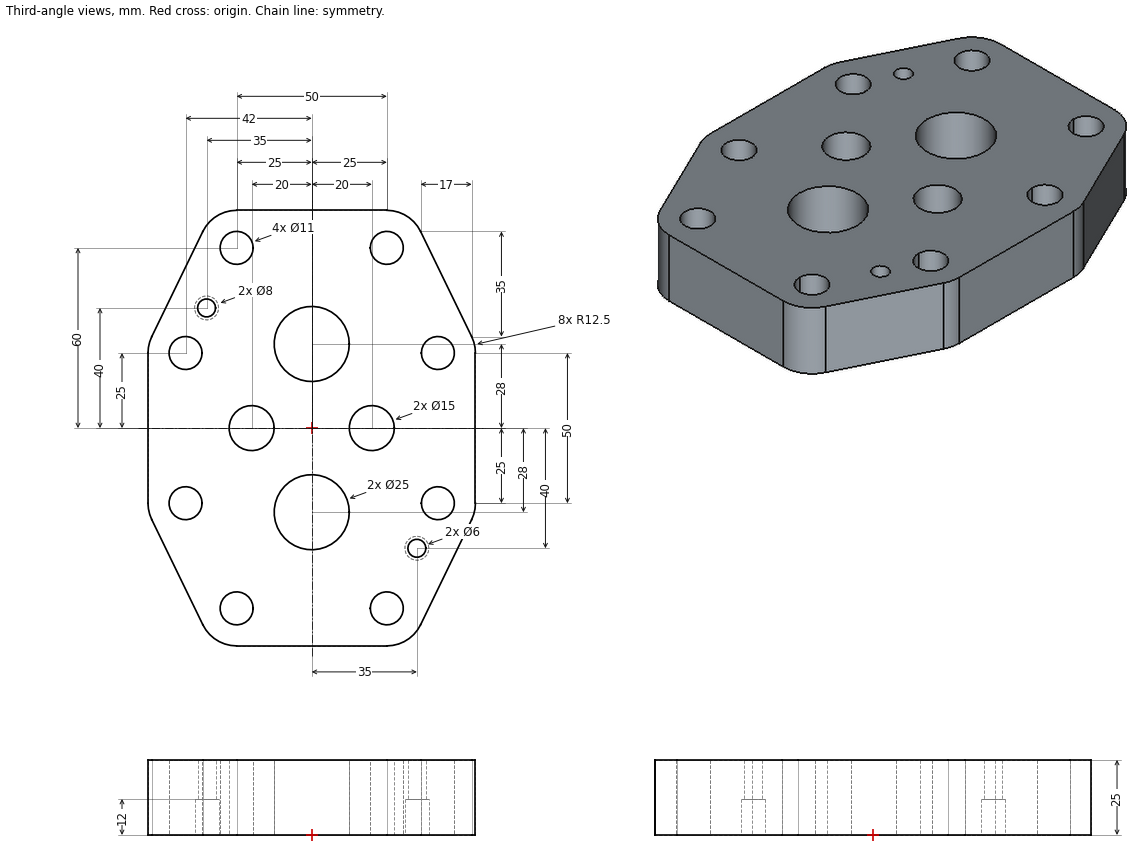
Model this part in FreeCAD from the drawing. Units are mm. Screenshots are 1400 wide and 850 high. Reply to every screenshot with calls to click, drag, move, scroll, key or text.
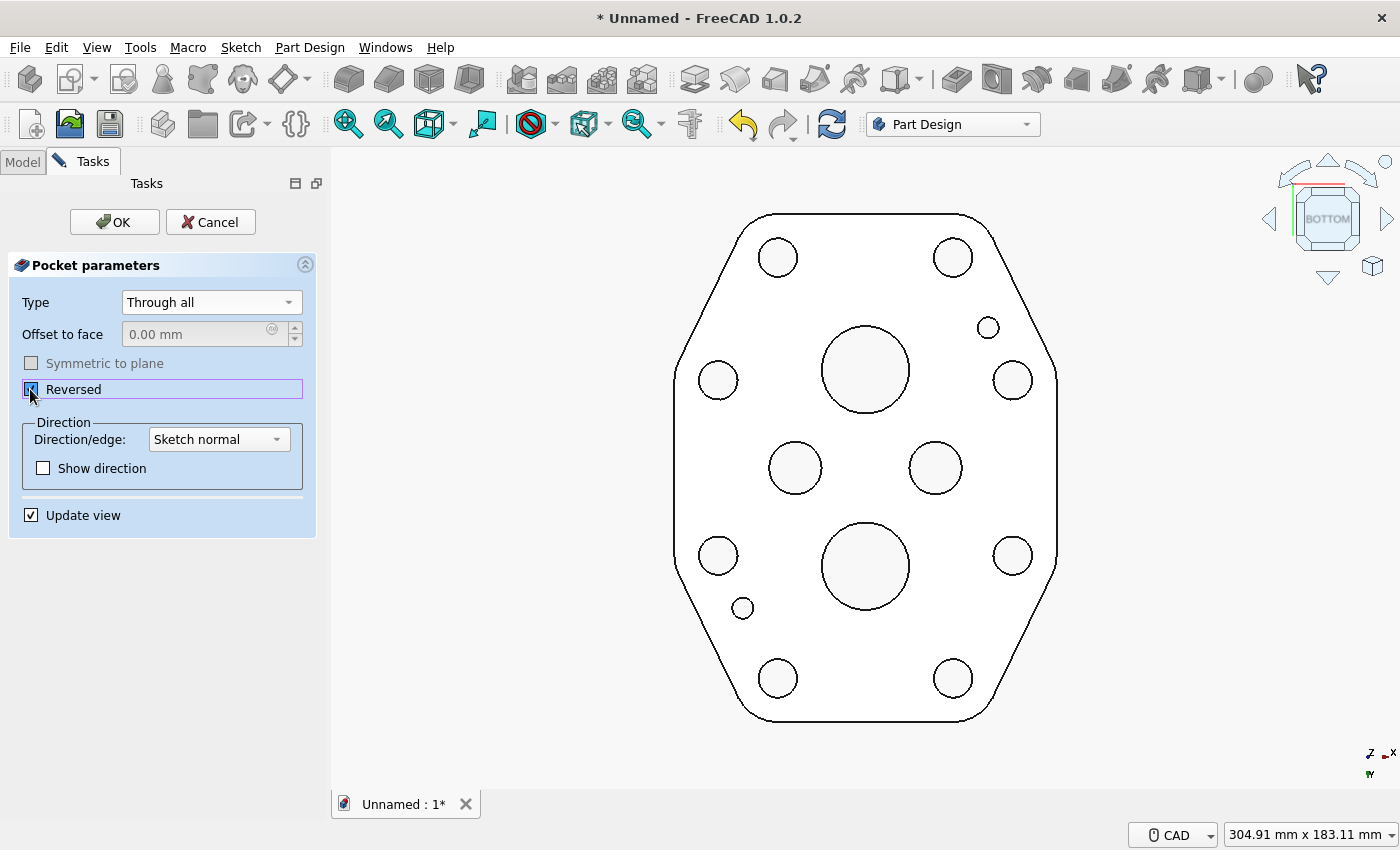
click(115, 222)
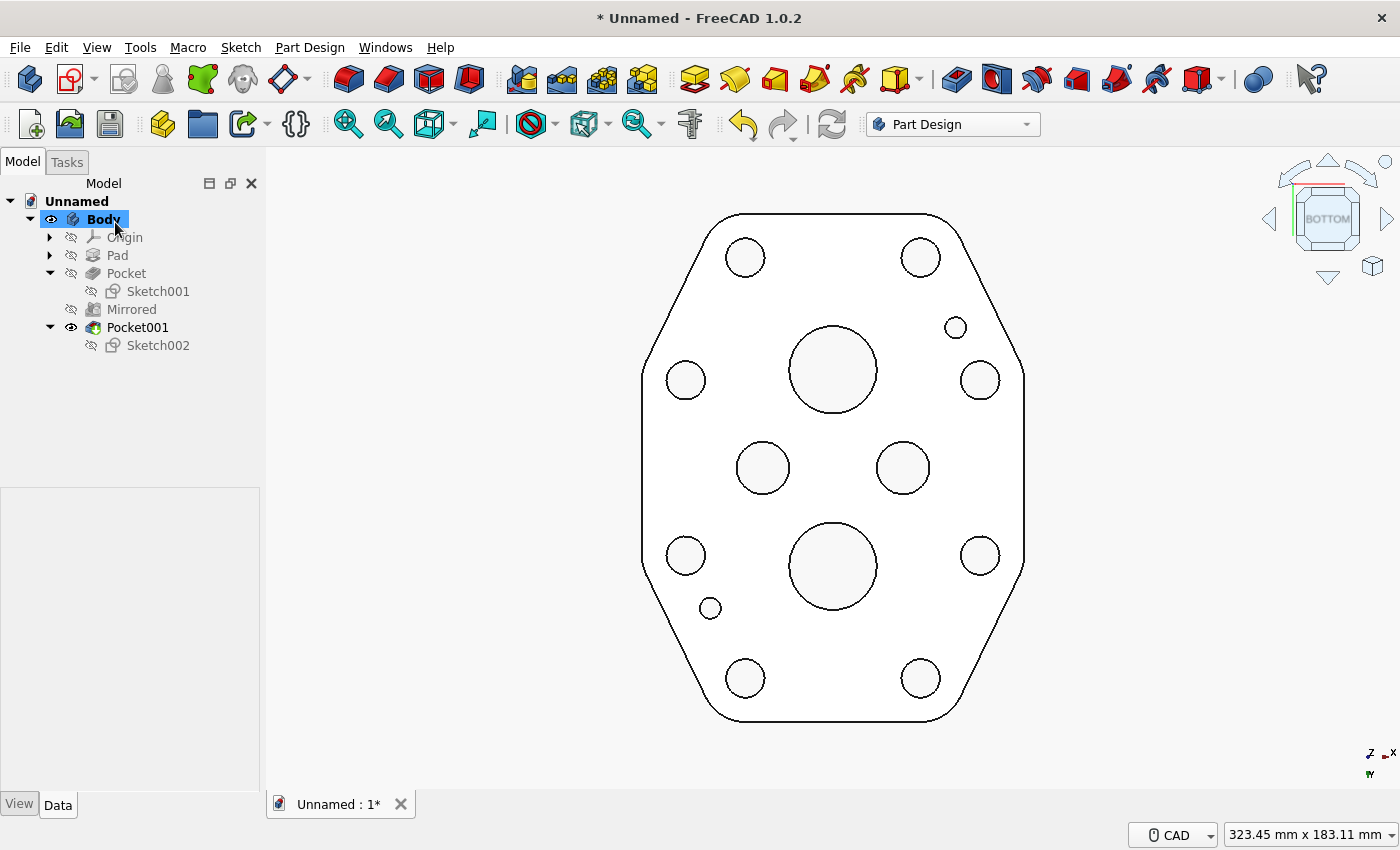
click(724, 322)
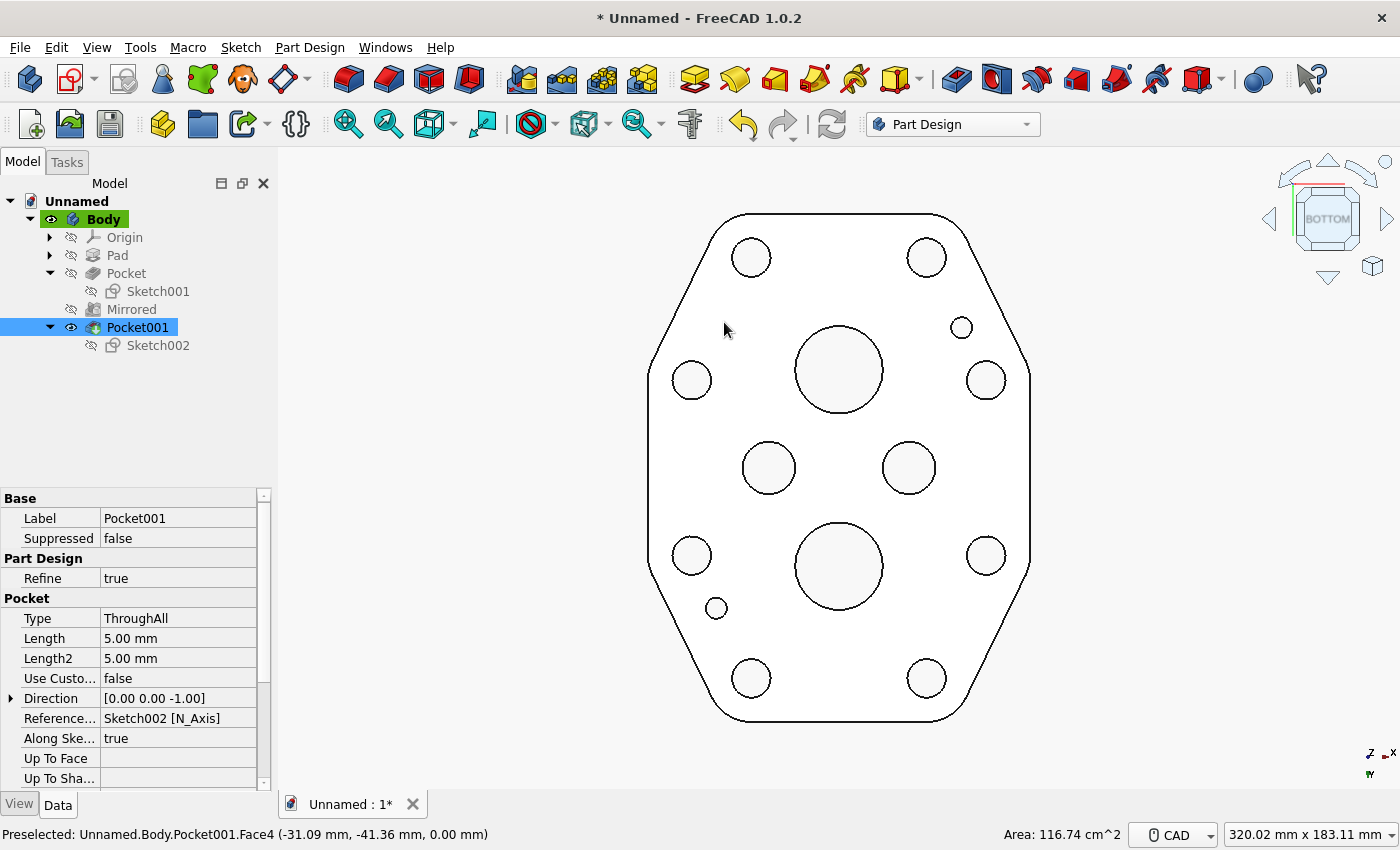
click(70, 80)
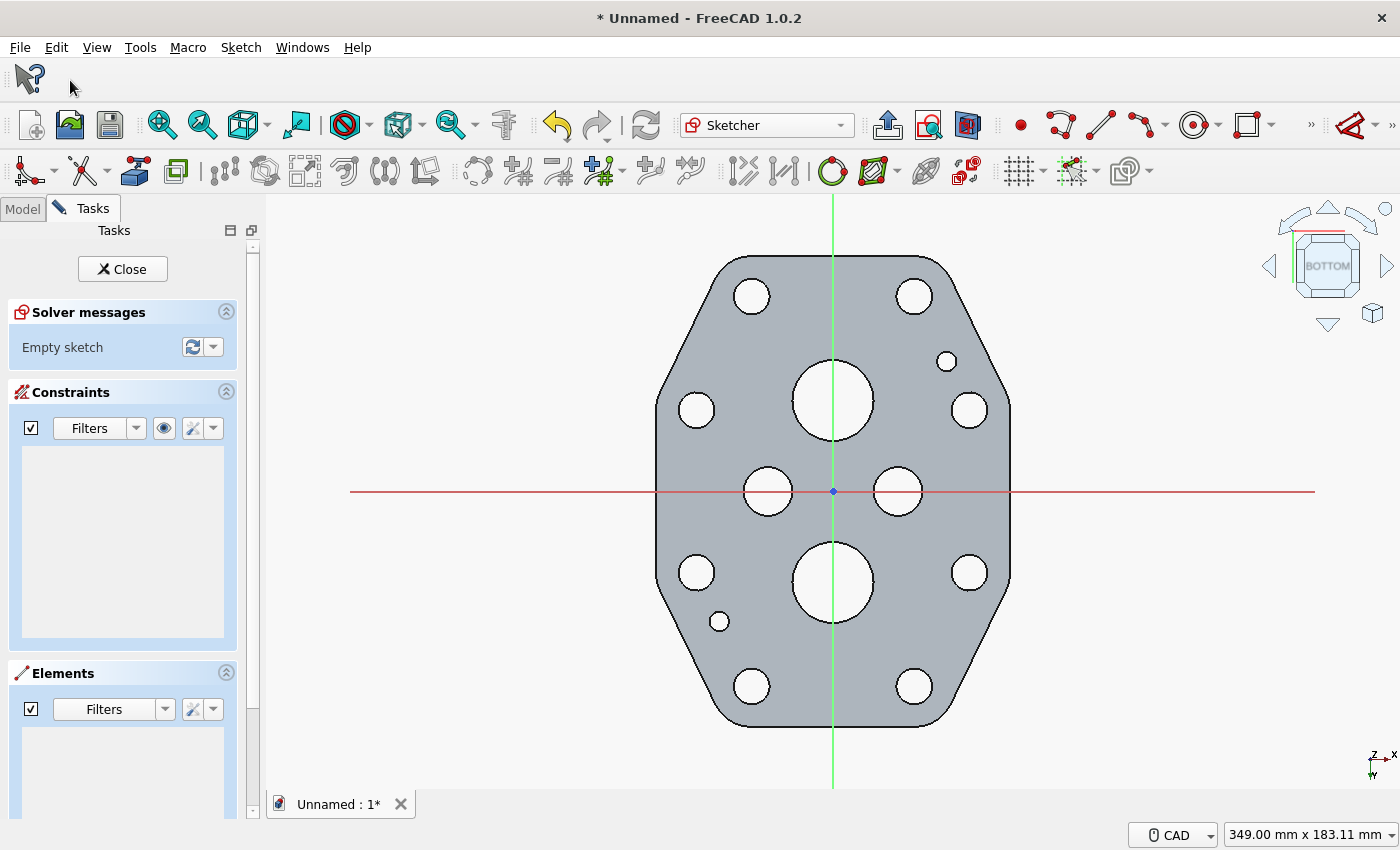
key(g)
key(c)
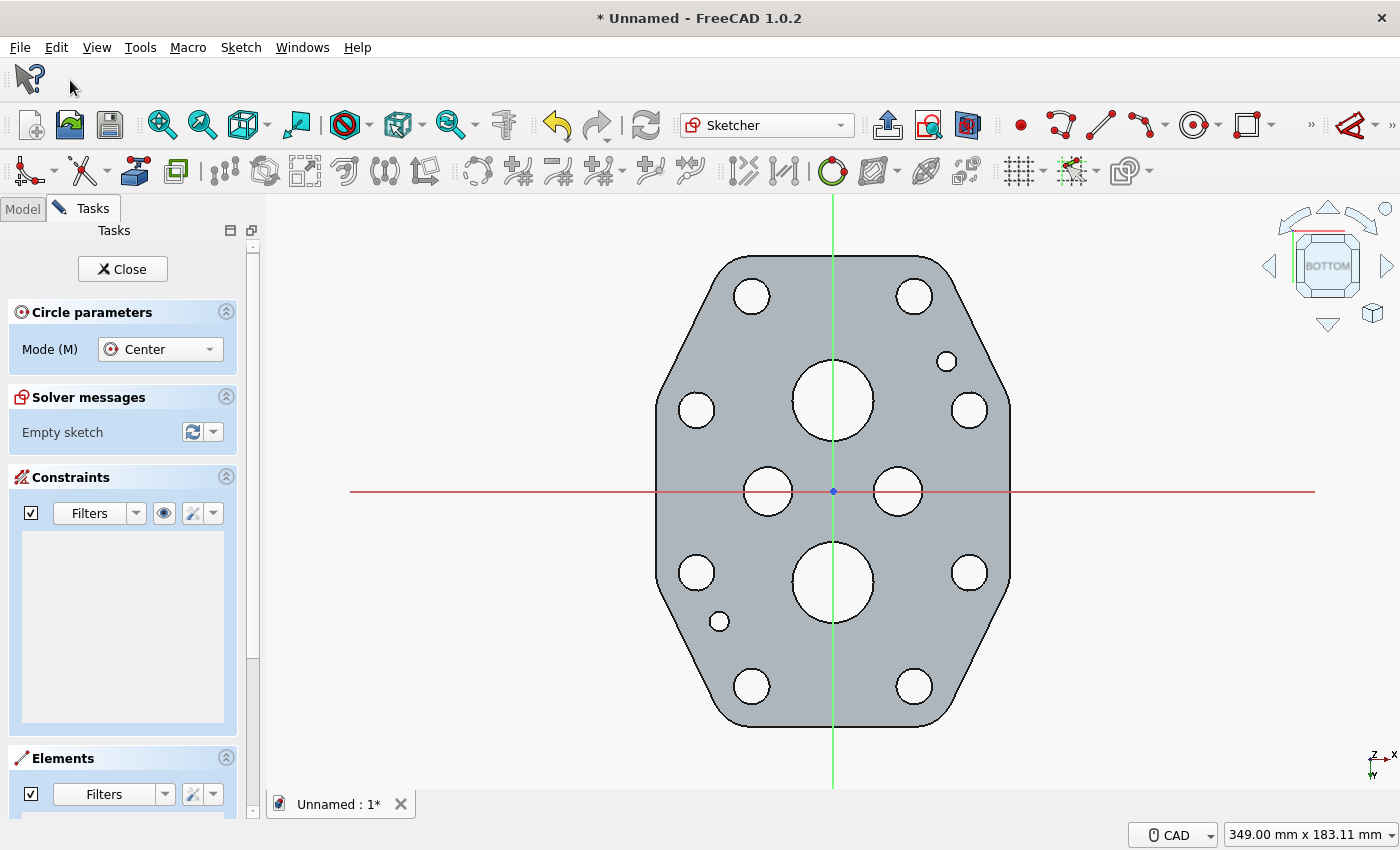
scroll(719, 621, up, 3)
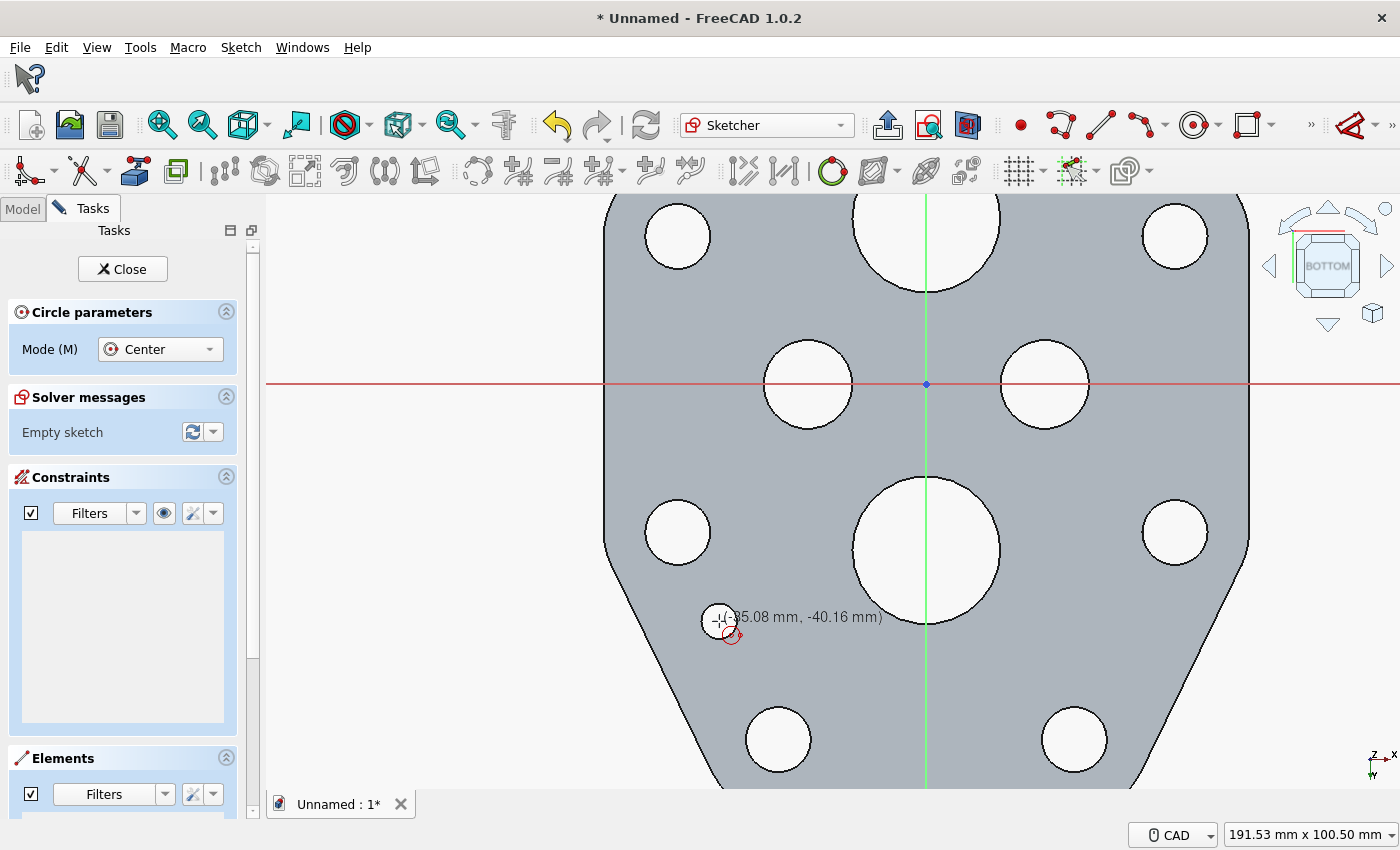
click(719, 621)
click(736, 605)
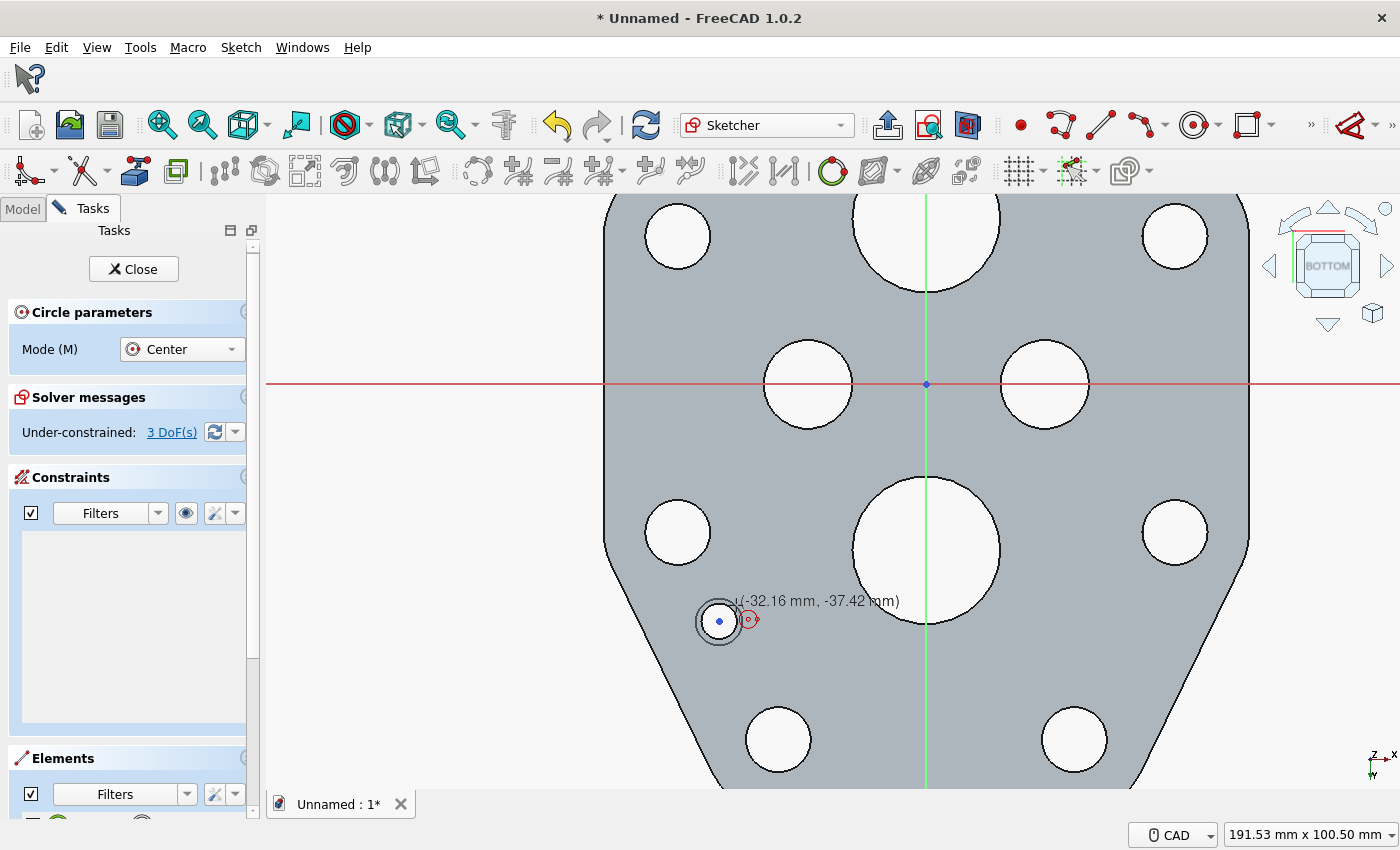
scroll(435, 709, down, 2)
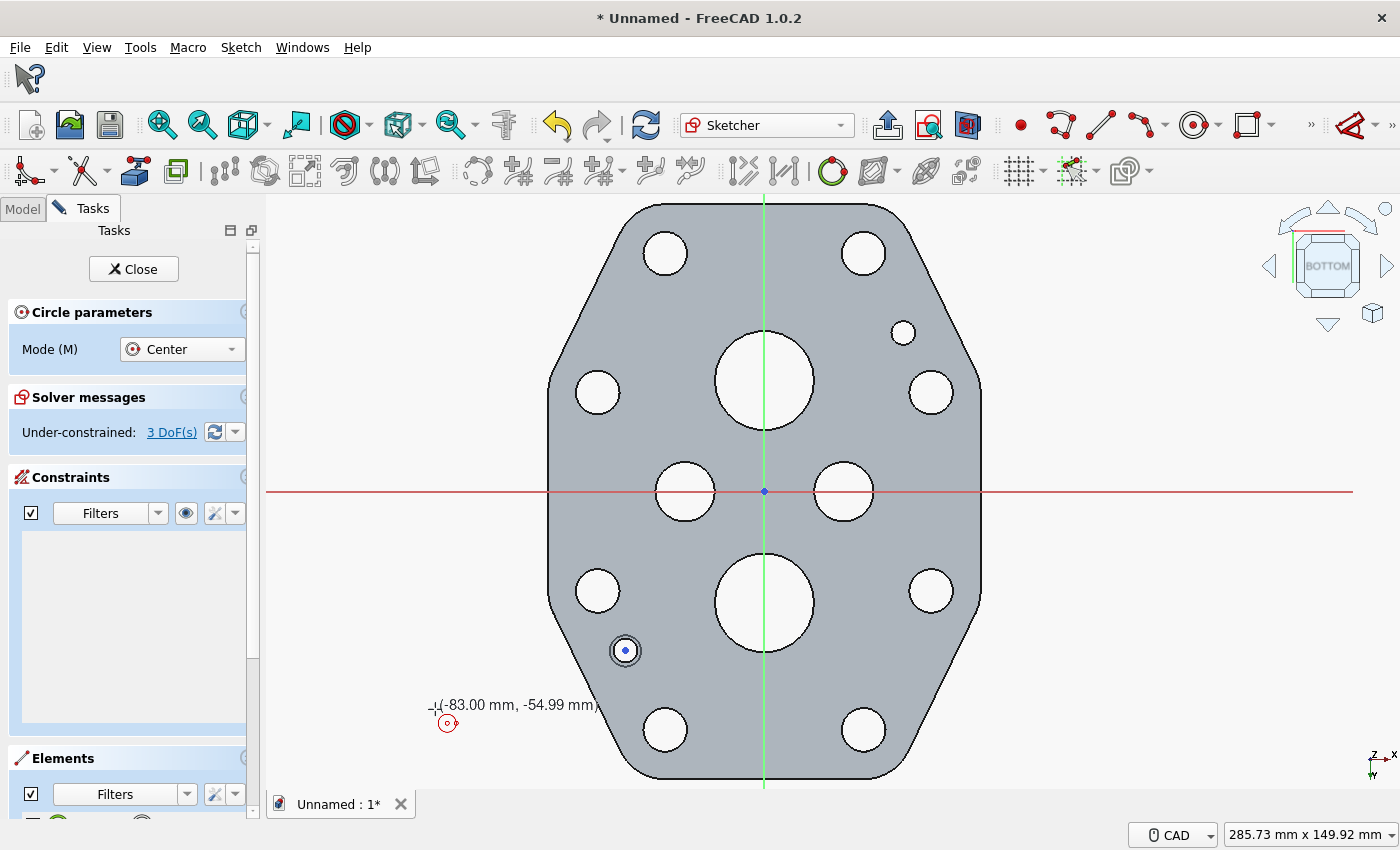
scroll(903, 333, up, 2)